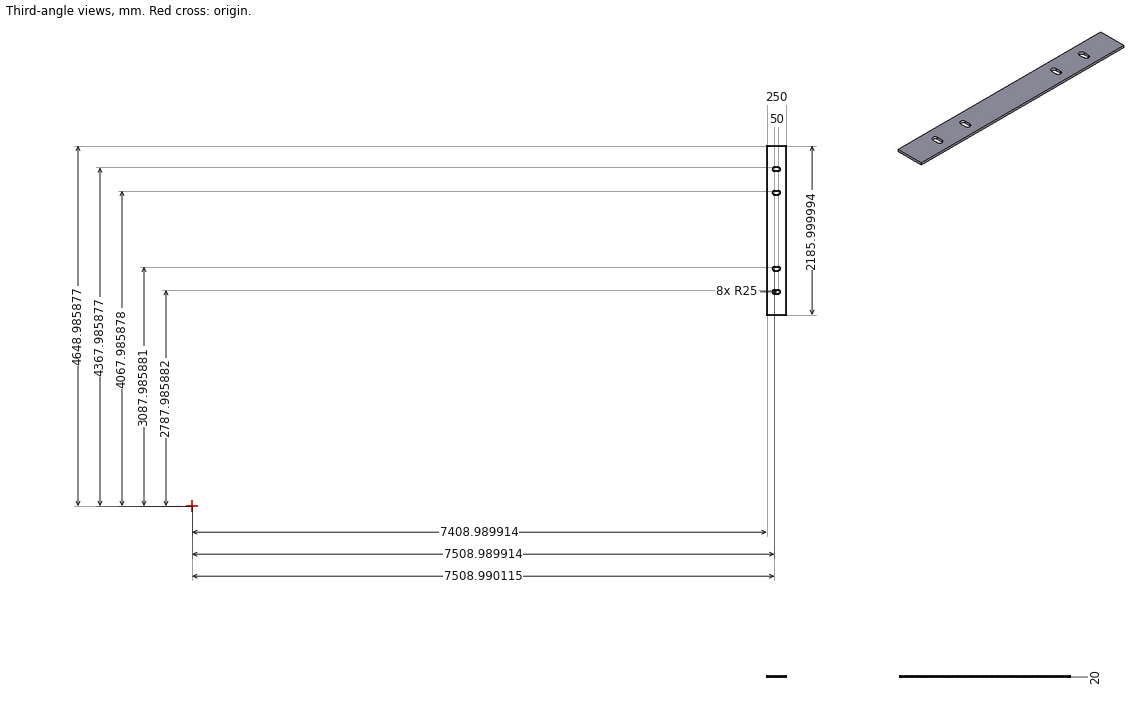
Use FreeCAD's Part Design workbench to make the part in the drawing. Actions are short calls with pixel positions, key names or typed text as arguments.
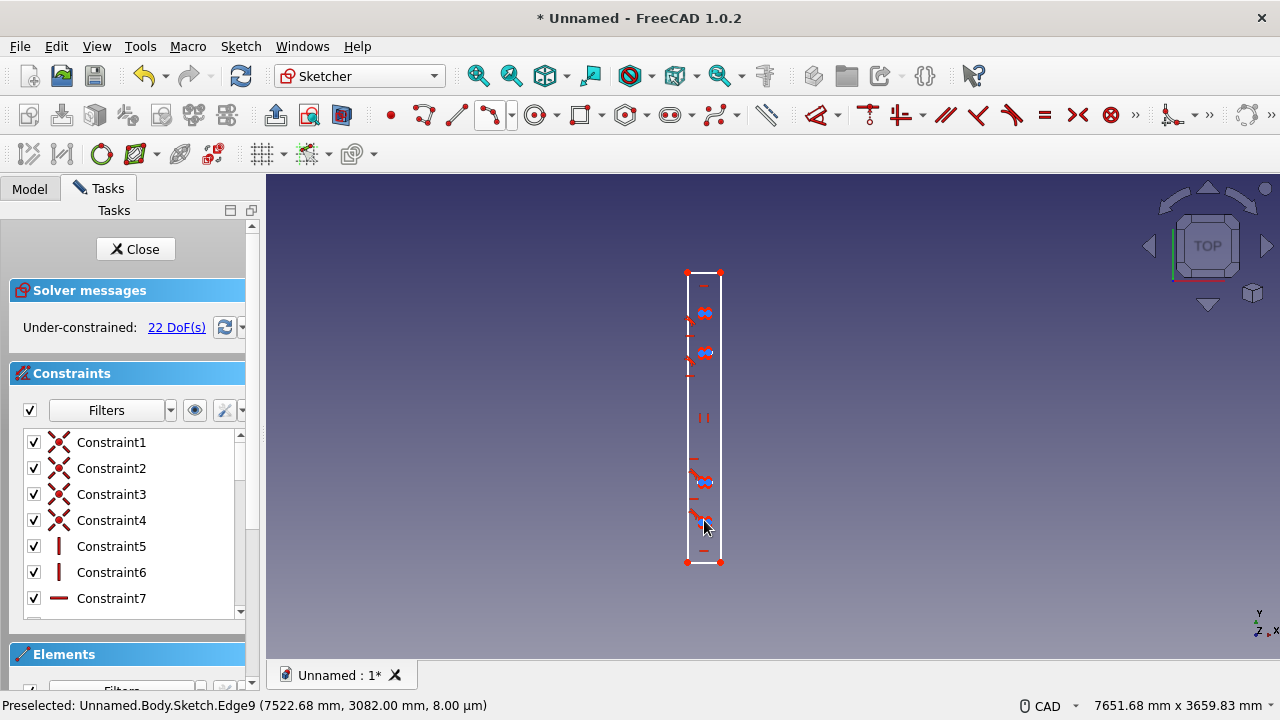
scroll(704, 311, up, 10)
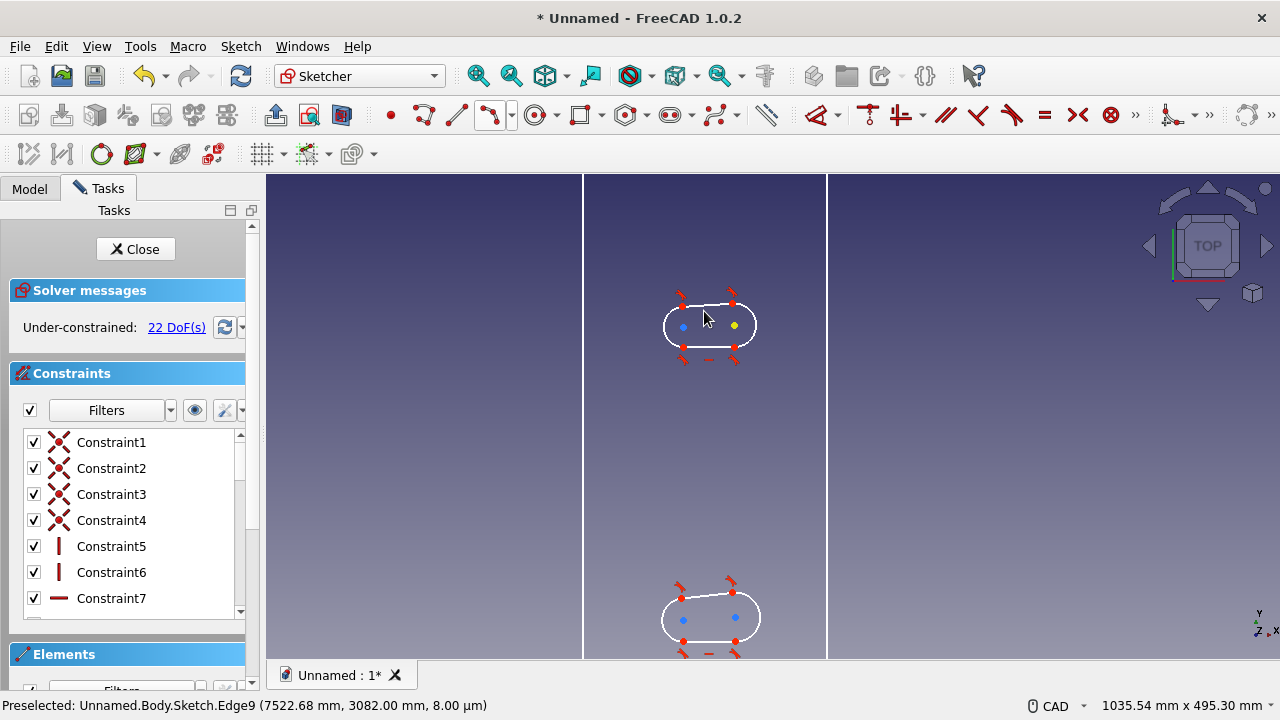
click(698, 306)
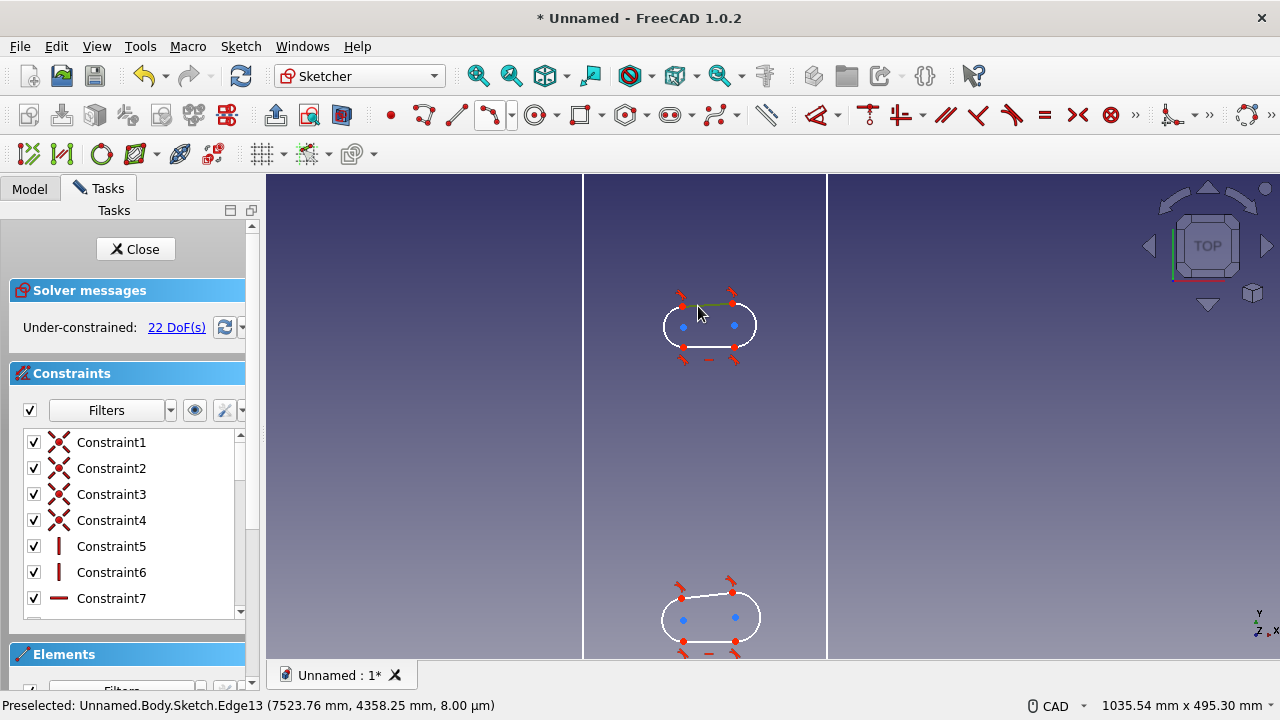
key(h)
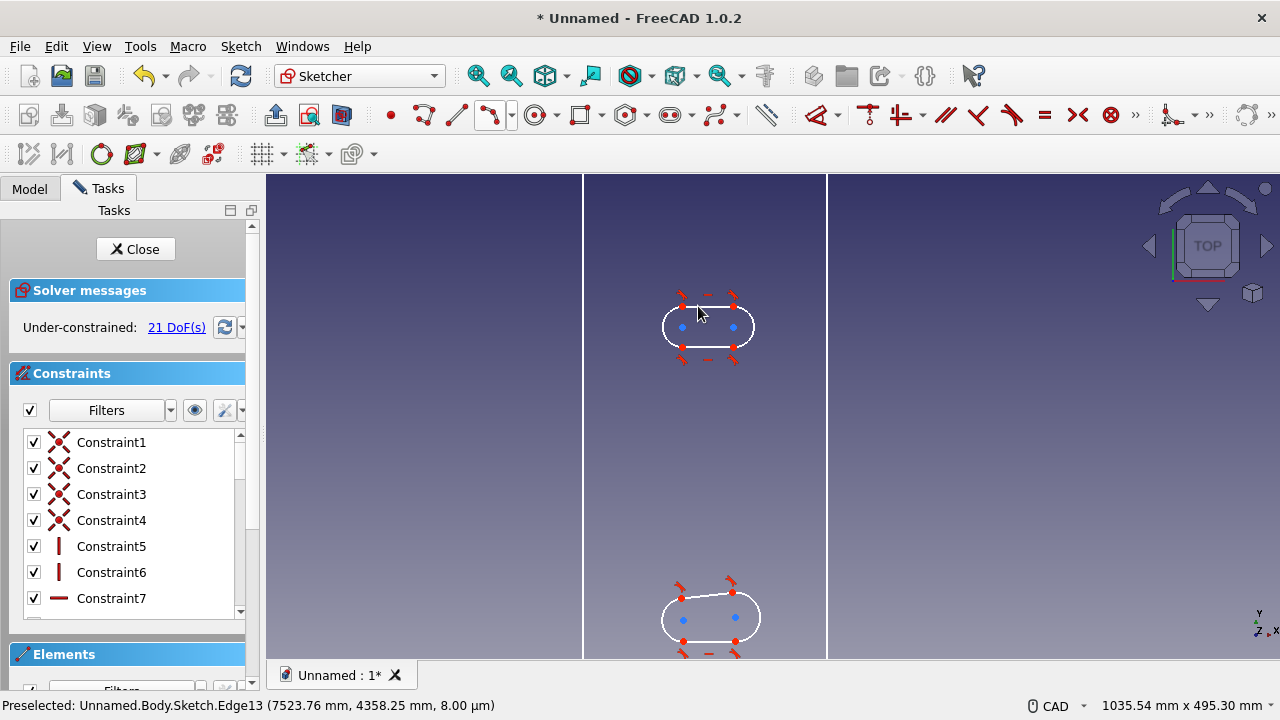
click(697, 597)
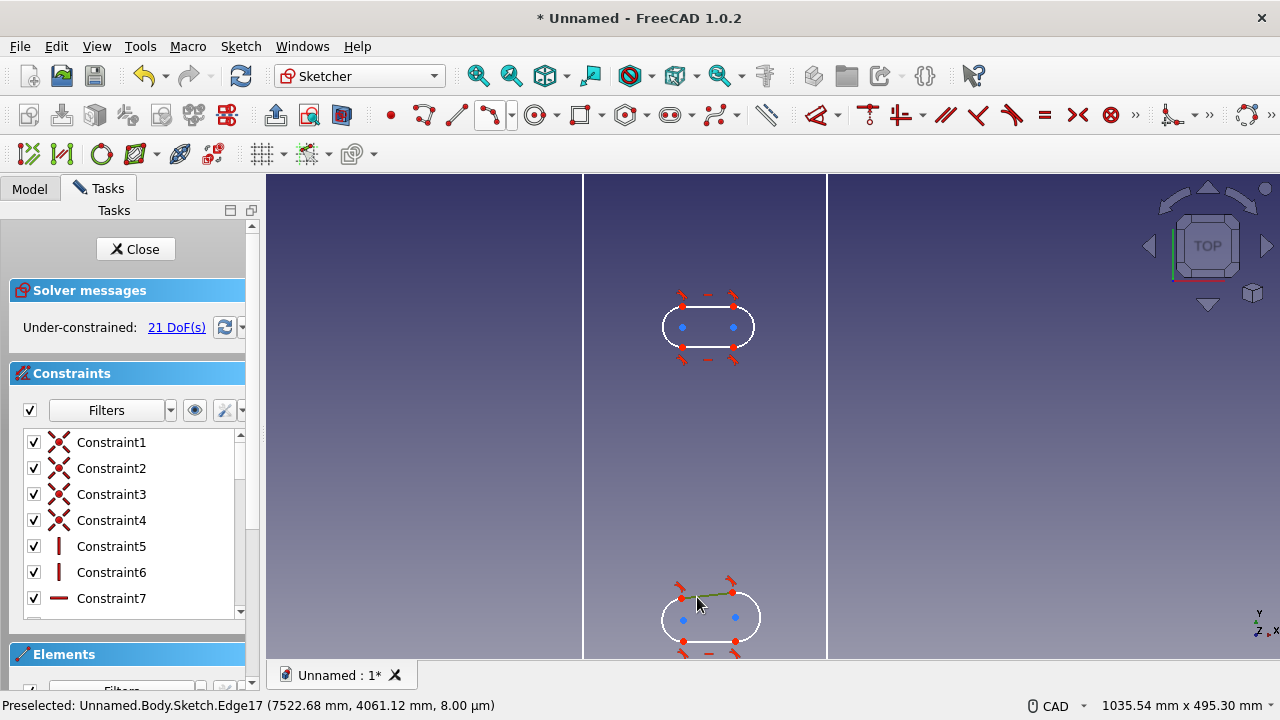
key(h)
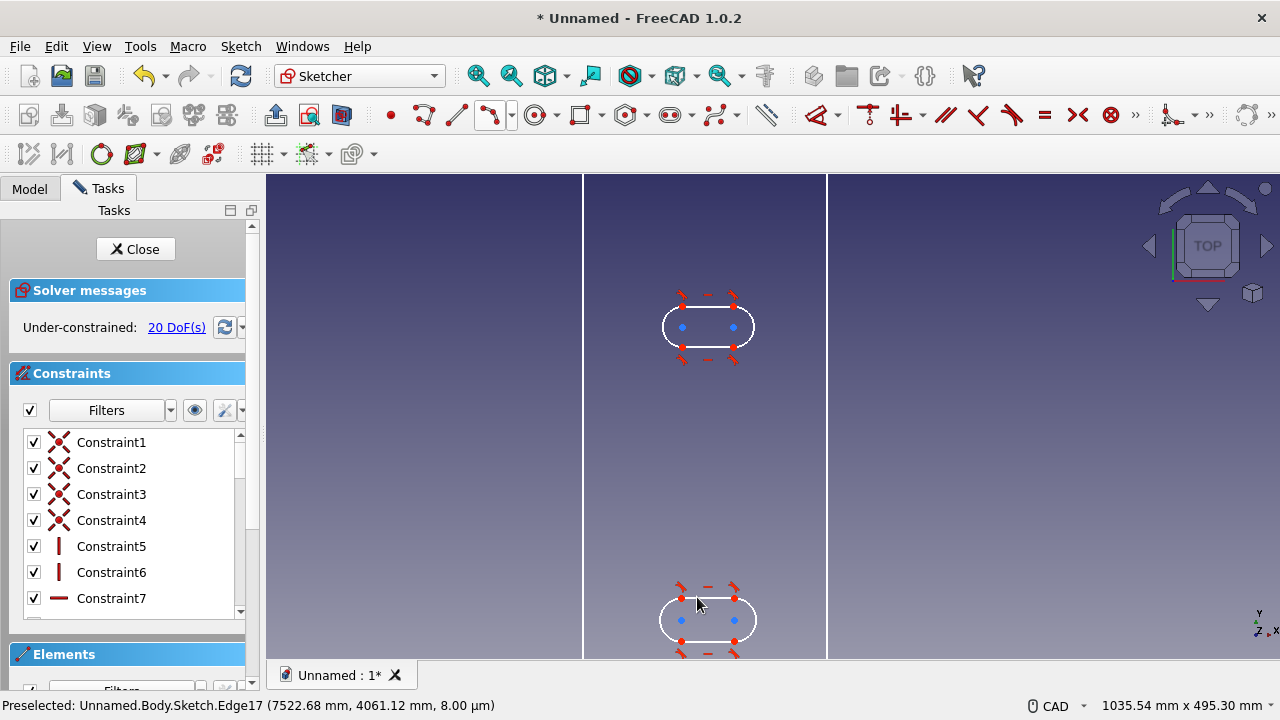
scroll(704, 311, down, 10)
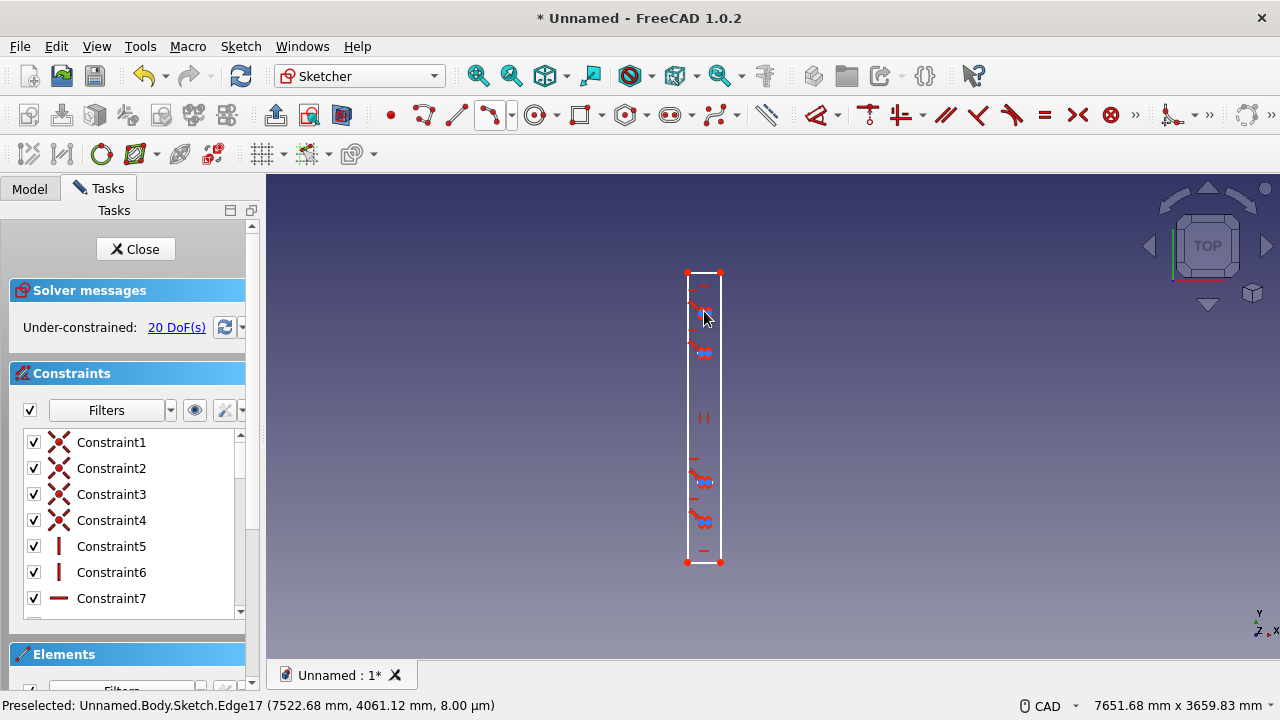
scroll(711, 524, up, 9)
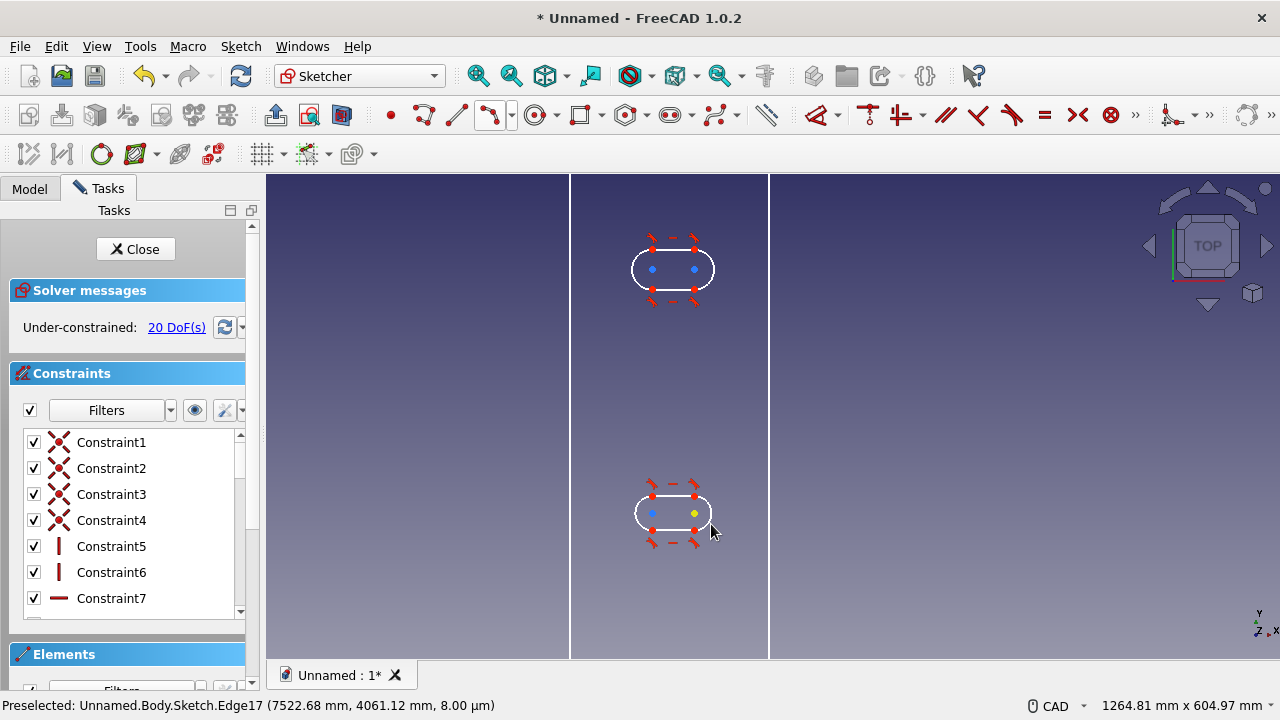
click(708, 523)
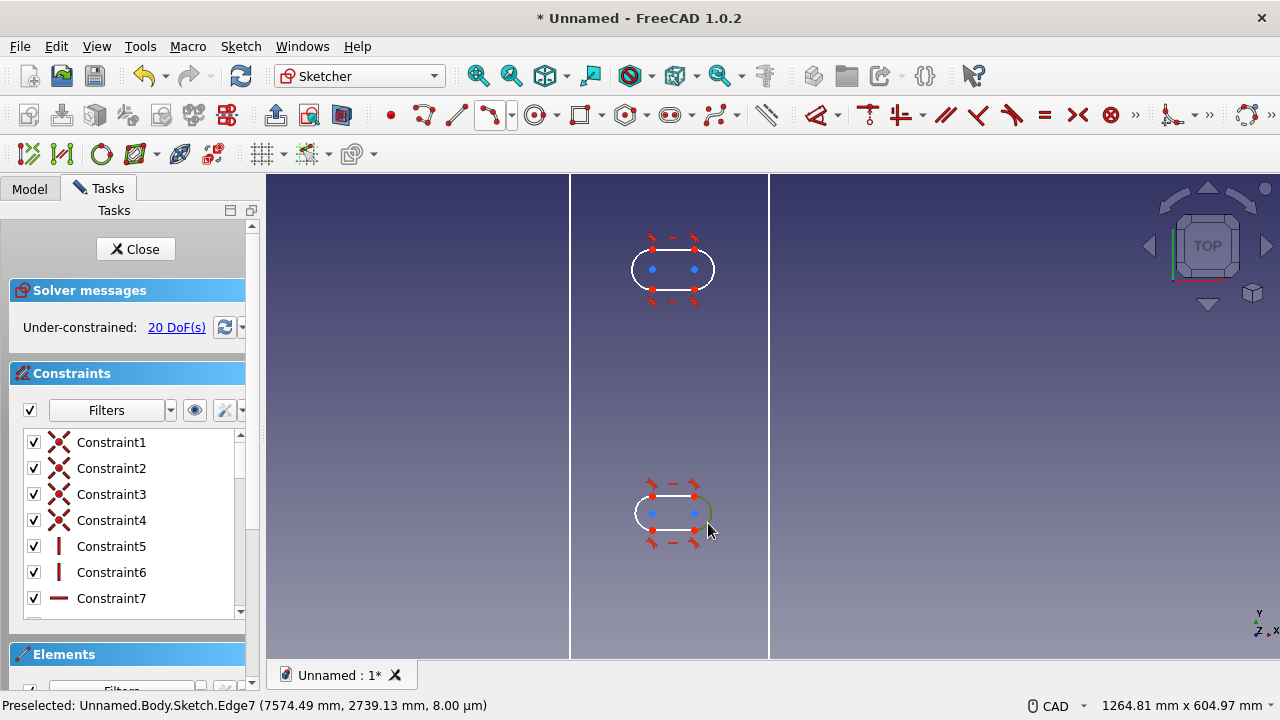
click(710, 282)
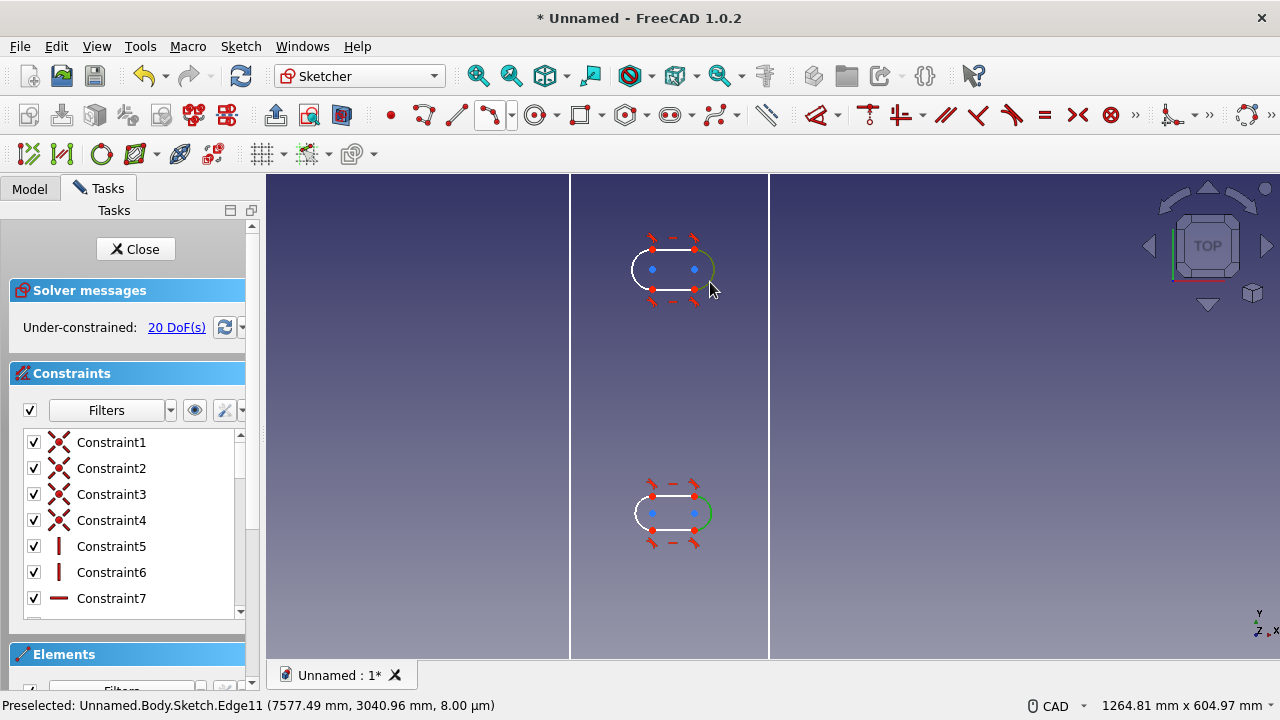
scroll(711, 524, down, 9)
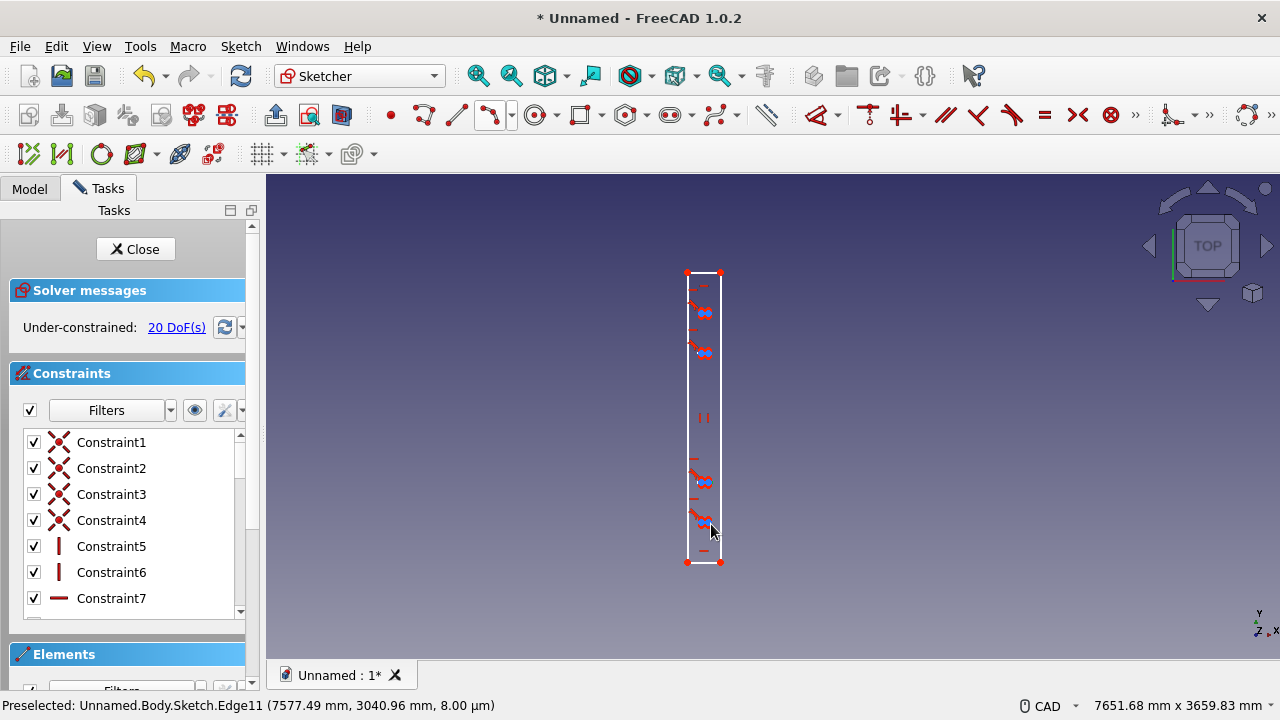
scroll(711, 315, up, 9)